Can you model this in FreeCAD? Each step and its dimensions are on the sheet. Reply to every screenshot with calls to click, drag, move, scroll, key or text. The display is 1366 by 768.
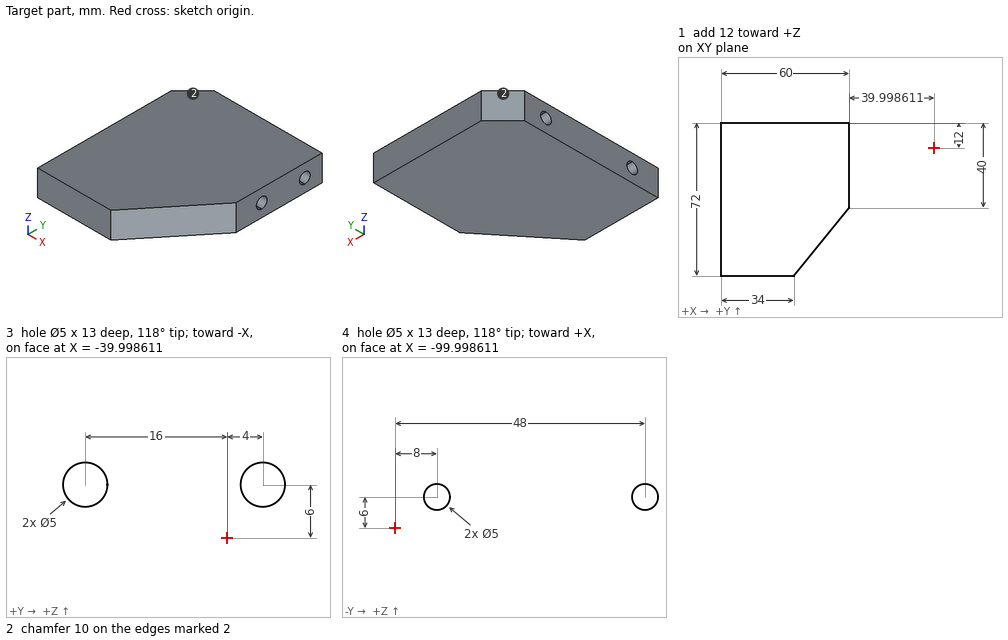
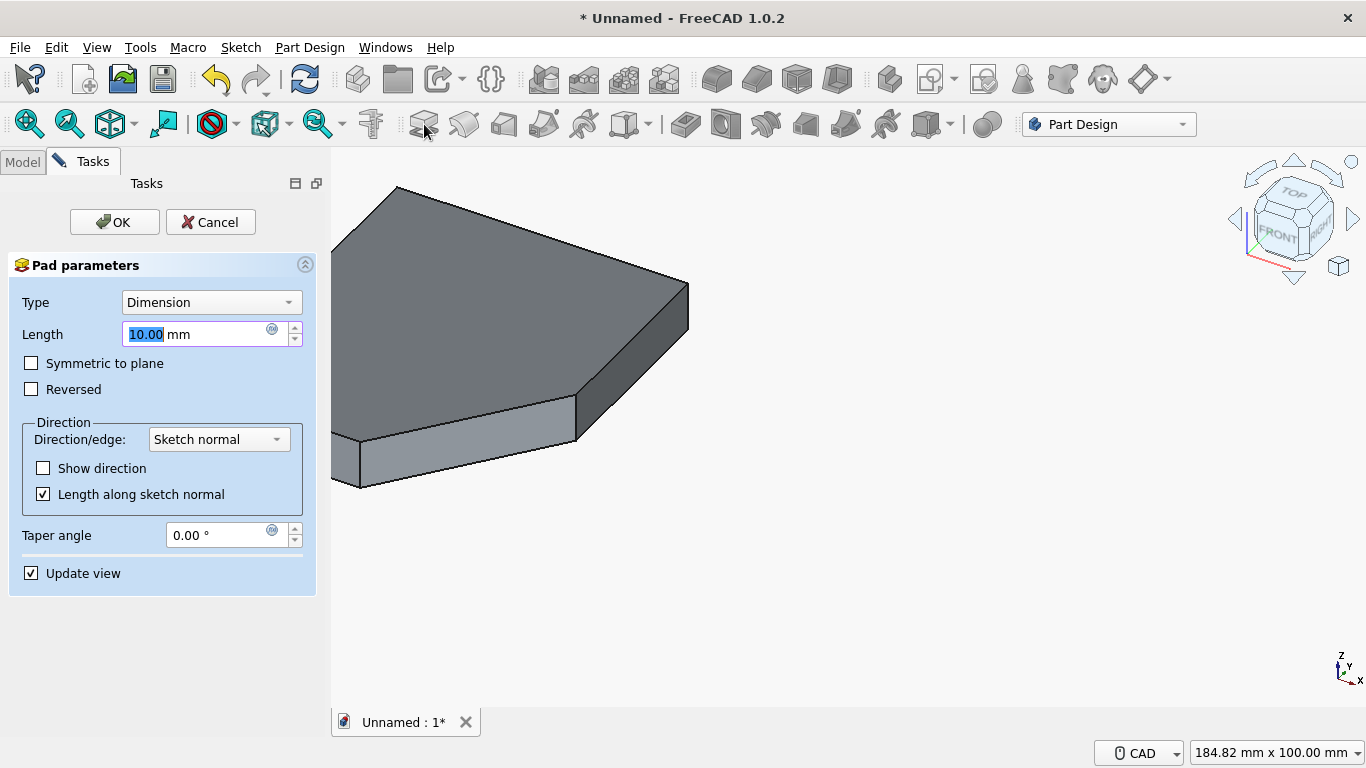
text(12)
key(Tab)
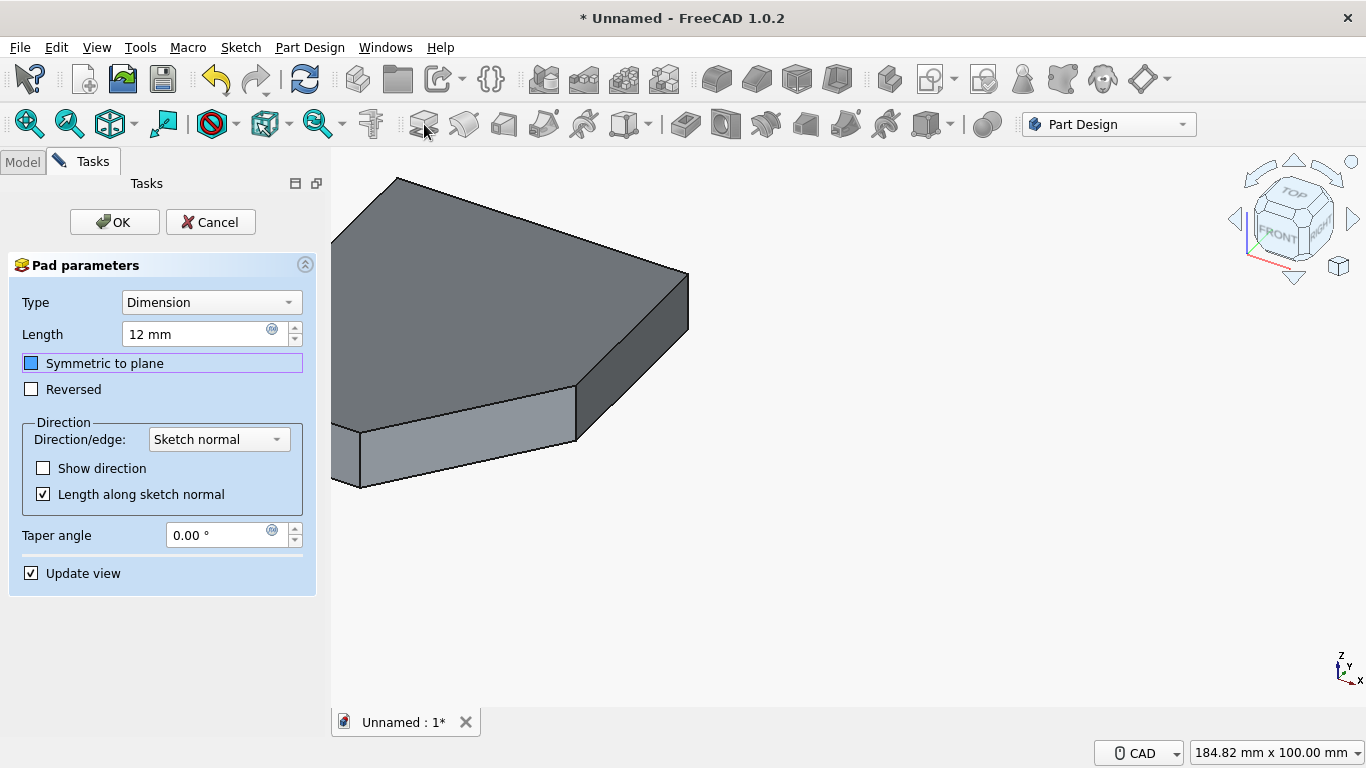
click(115, 222)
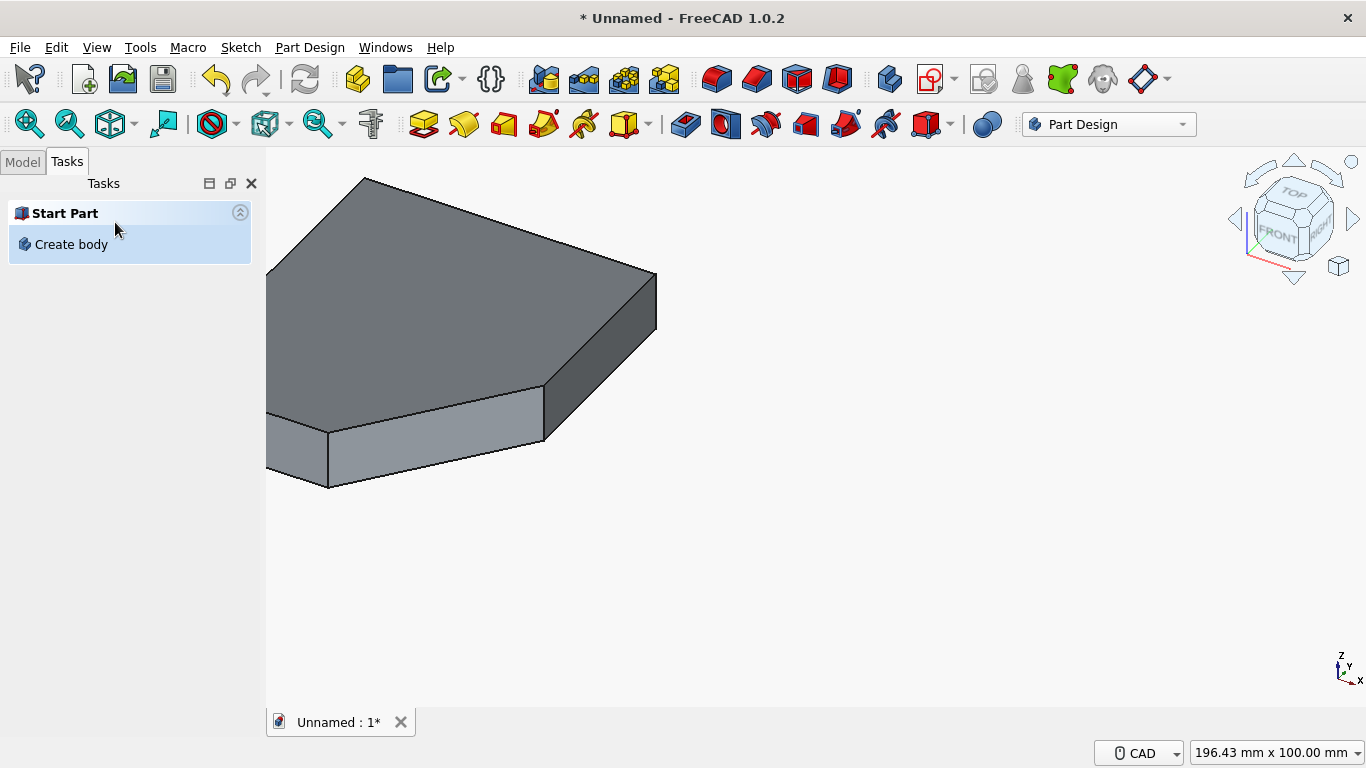
click(30, 124)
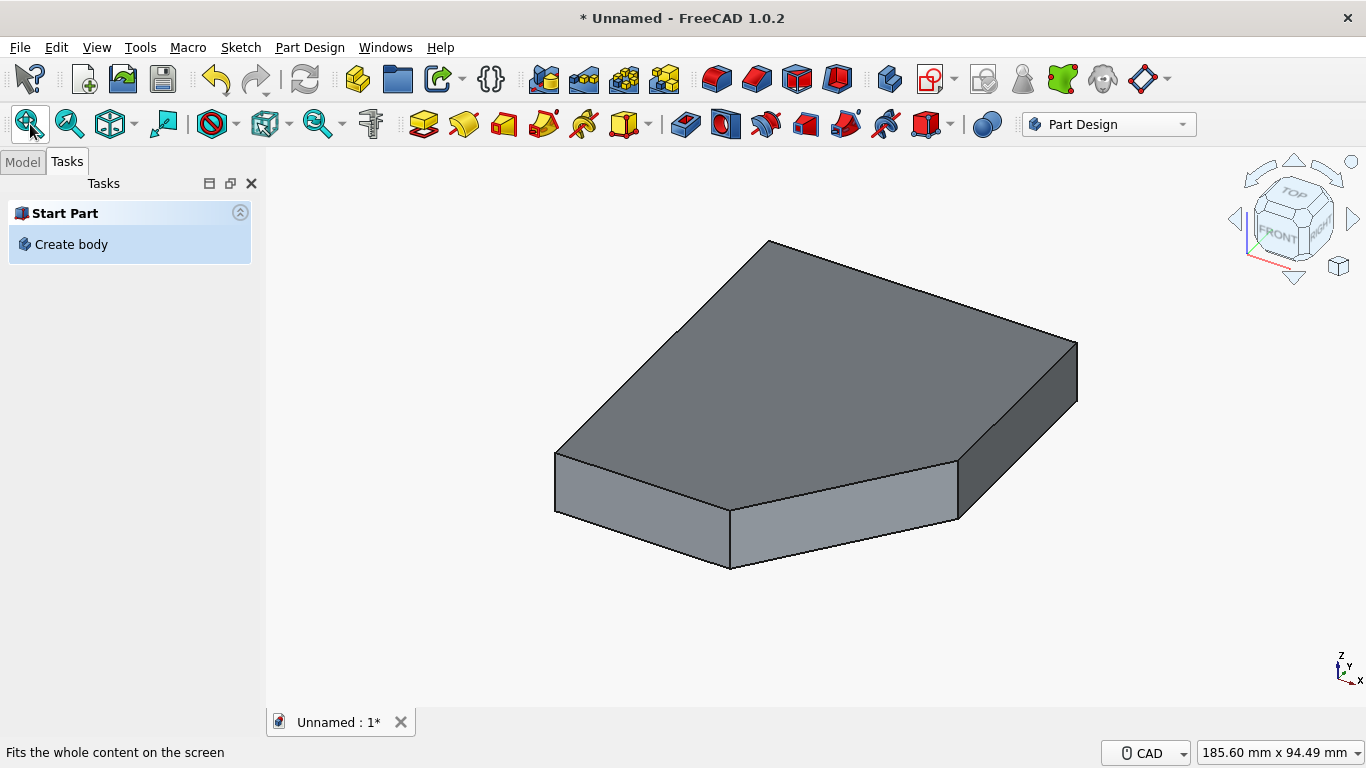
key(0)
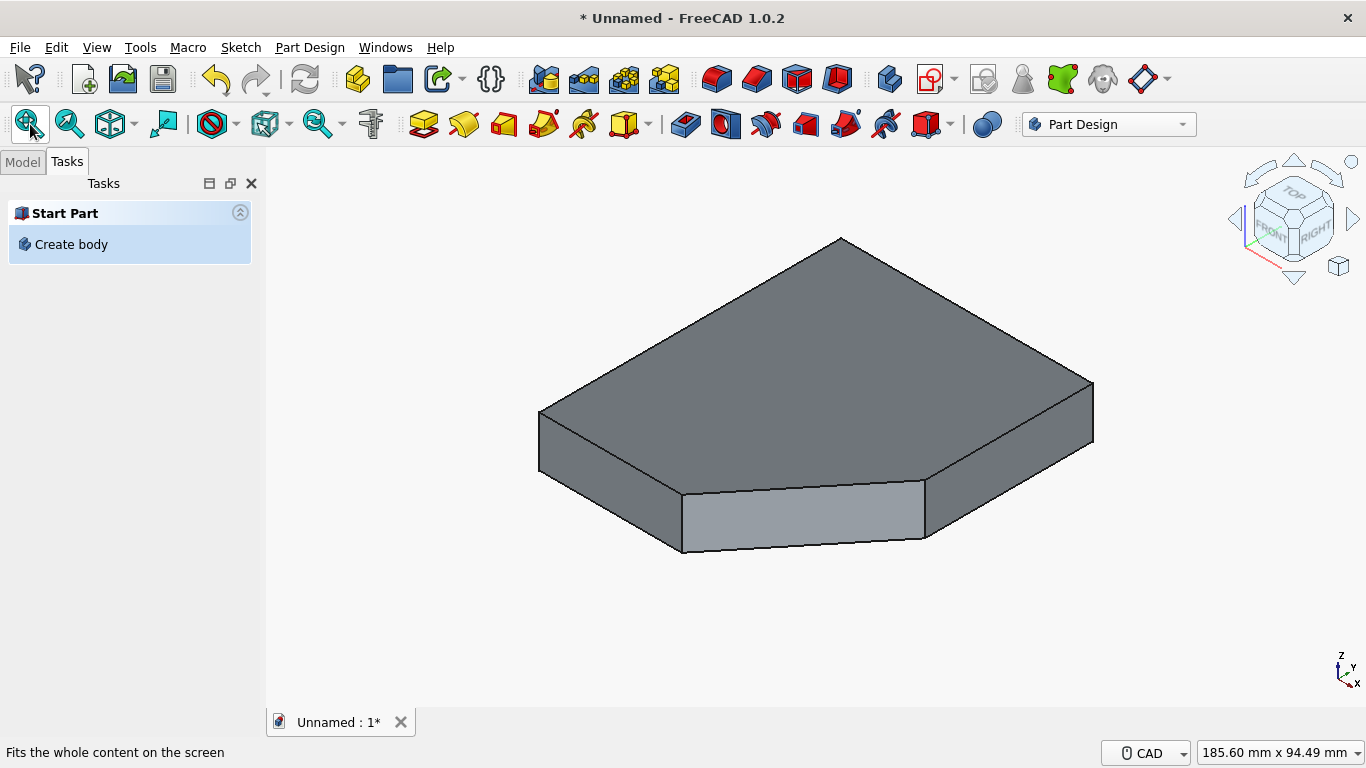
key(2)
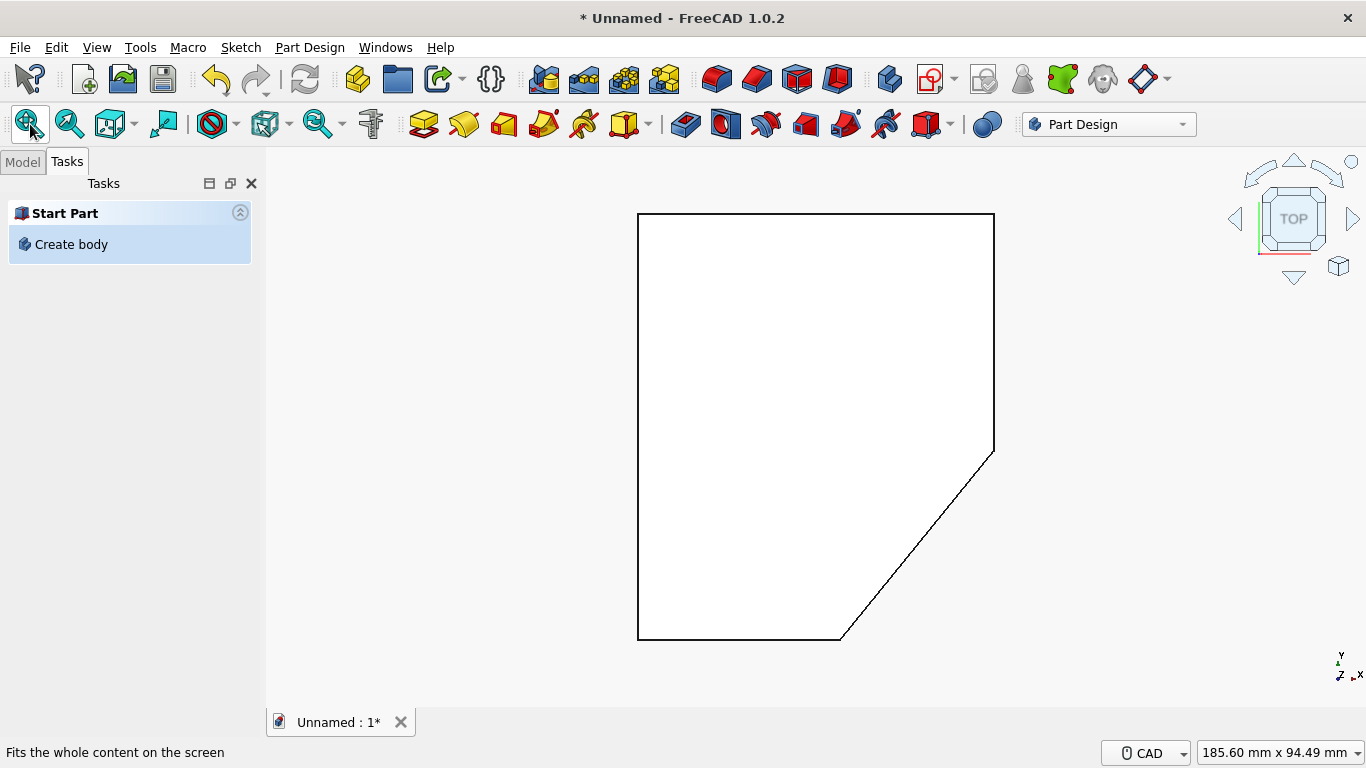
key(1)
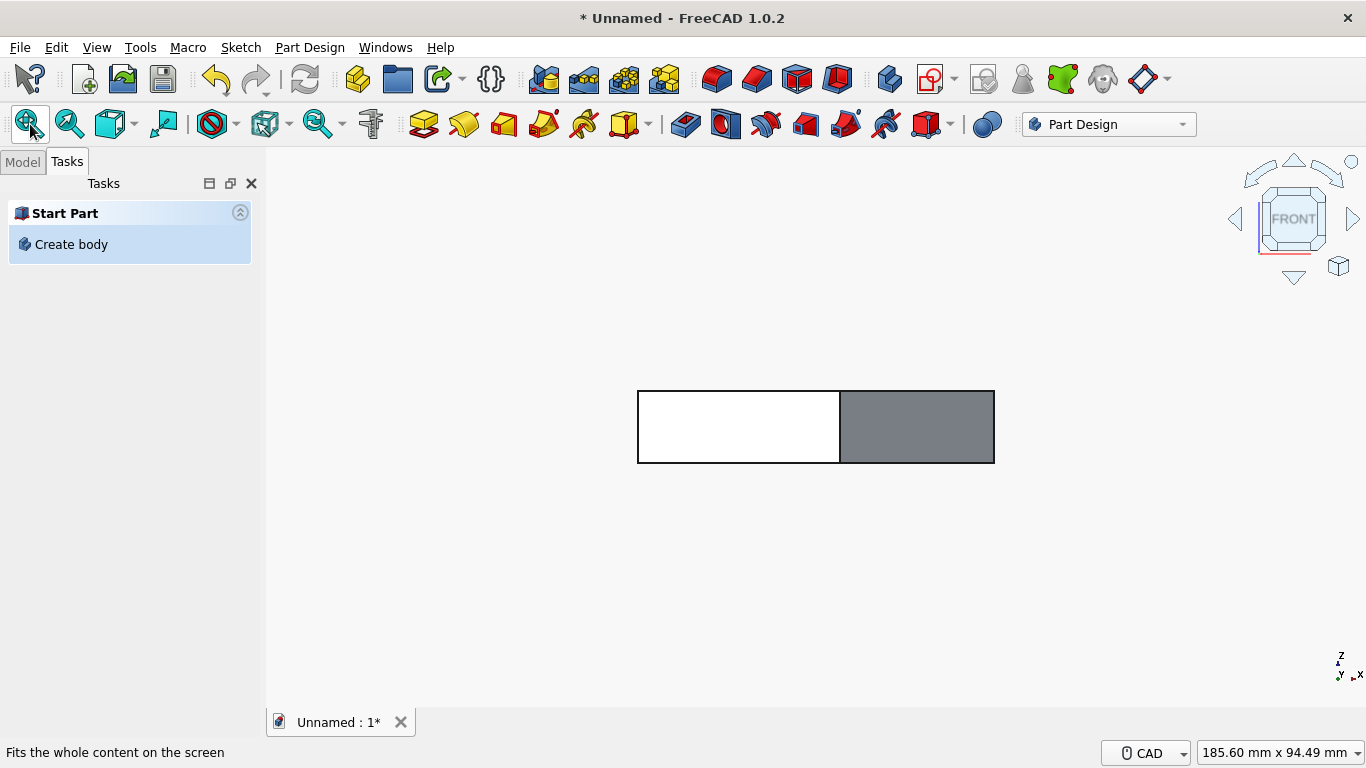
click(30, 124)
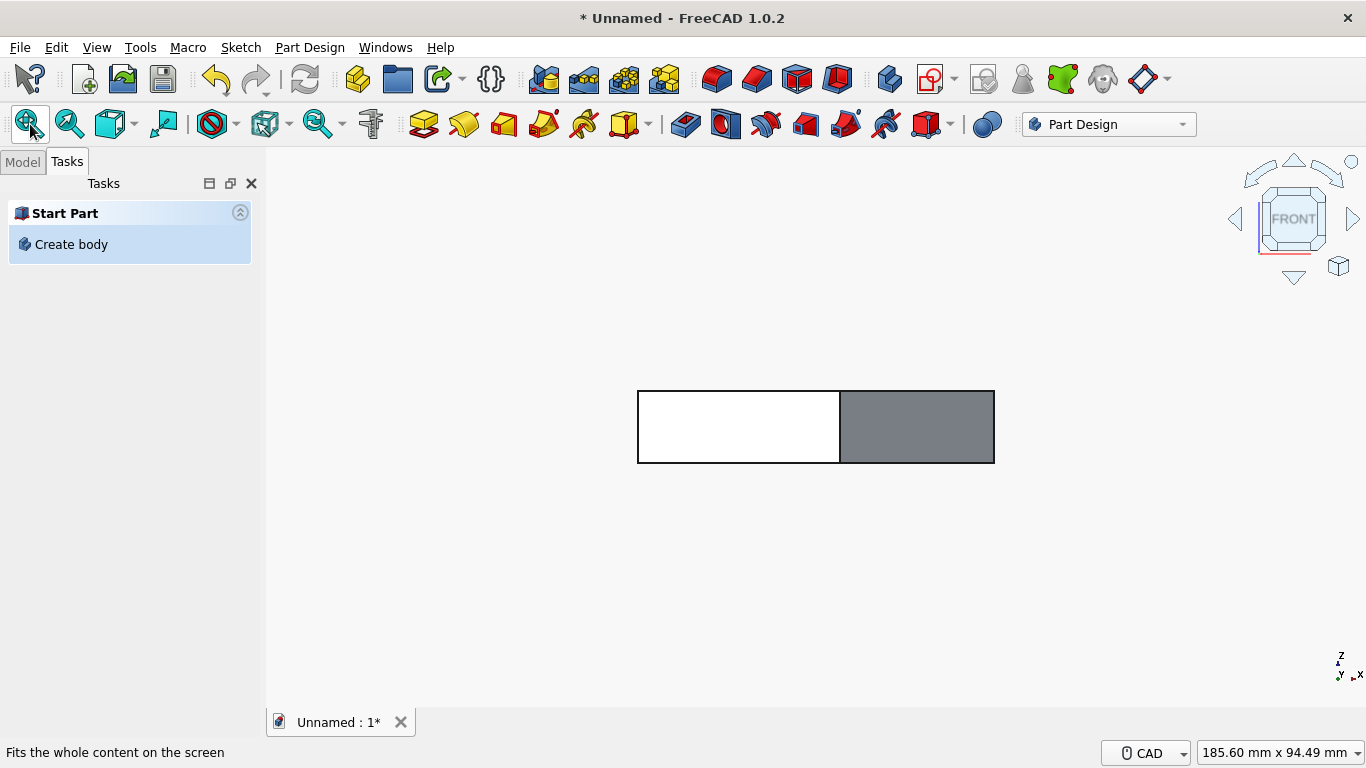
key(3)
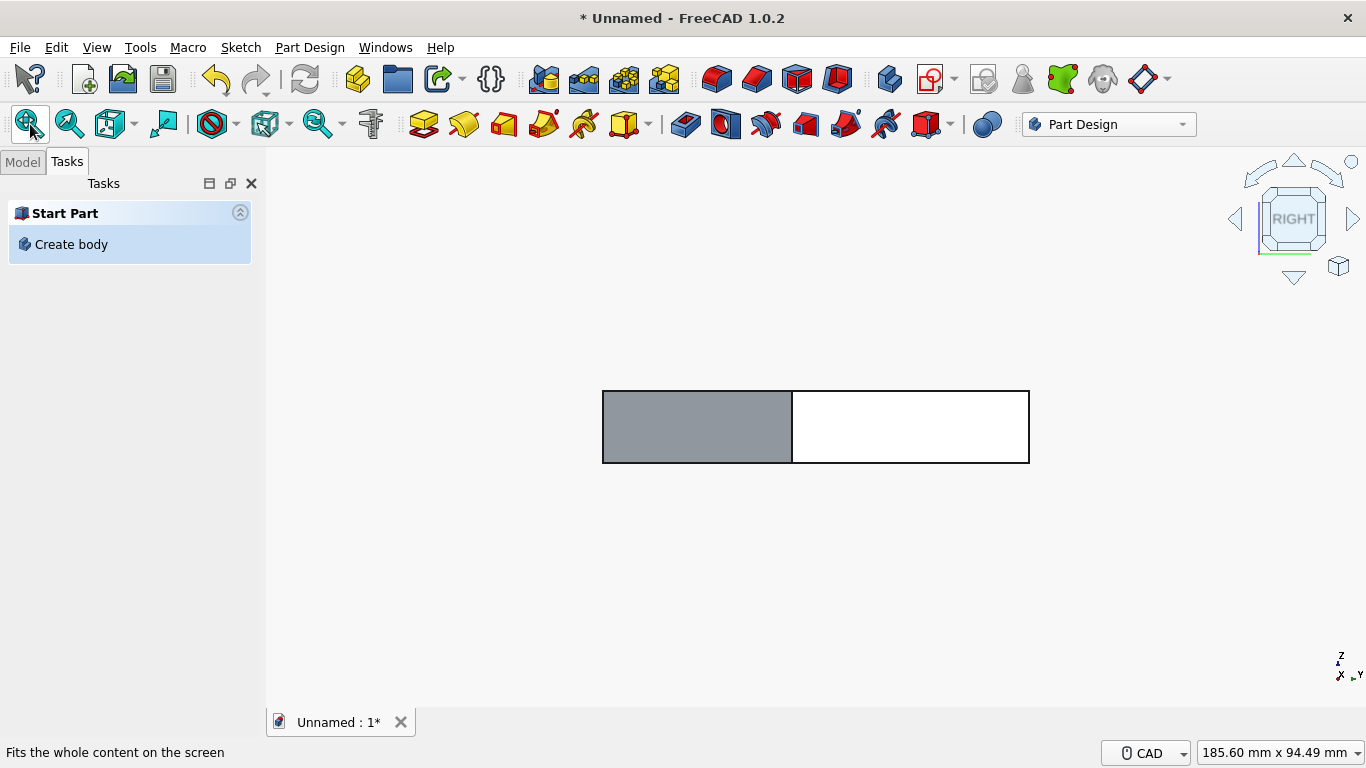
click(30, 124)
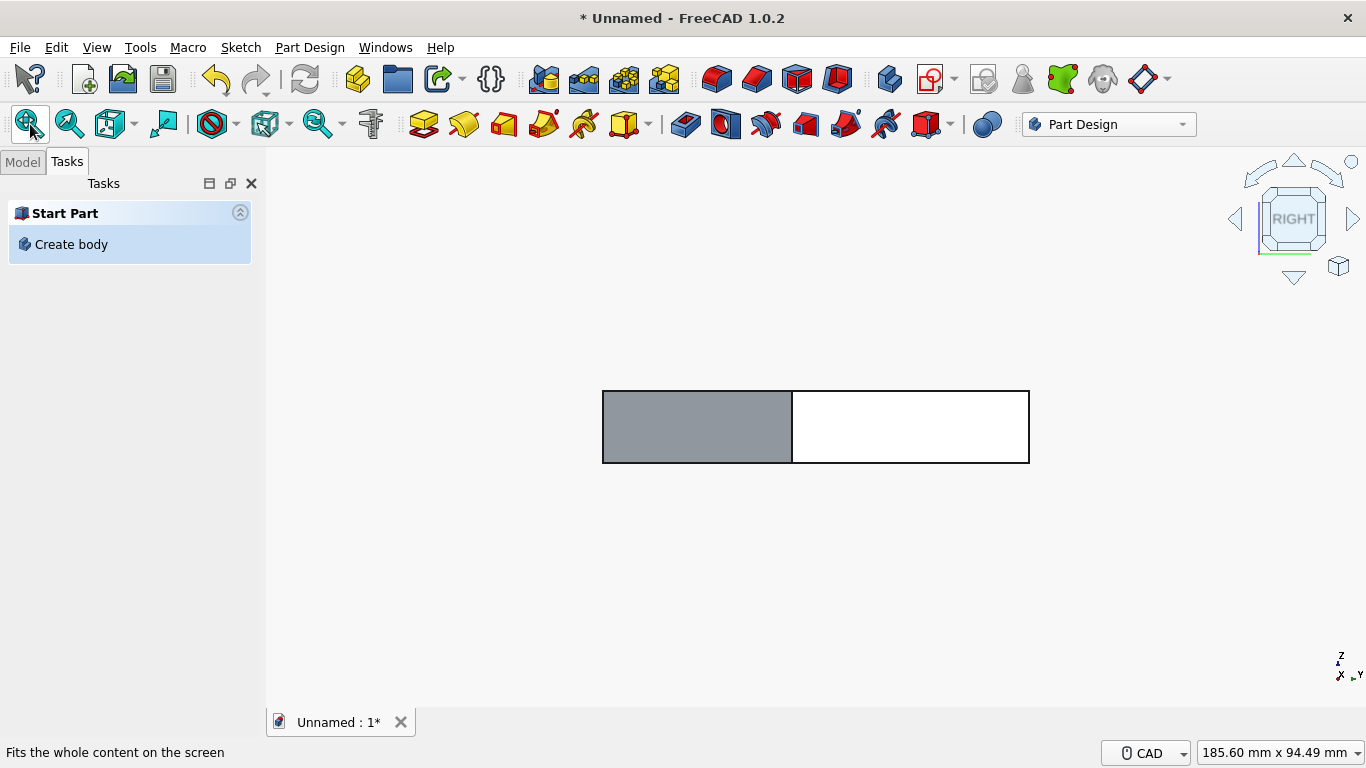
key(5)